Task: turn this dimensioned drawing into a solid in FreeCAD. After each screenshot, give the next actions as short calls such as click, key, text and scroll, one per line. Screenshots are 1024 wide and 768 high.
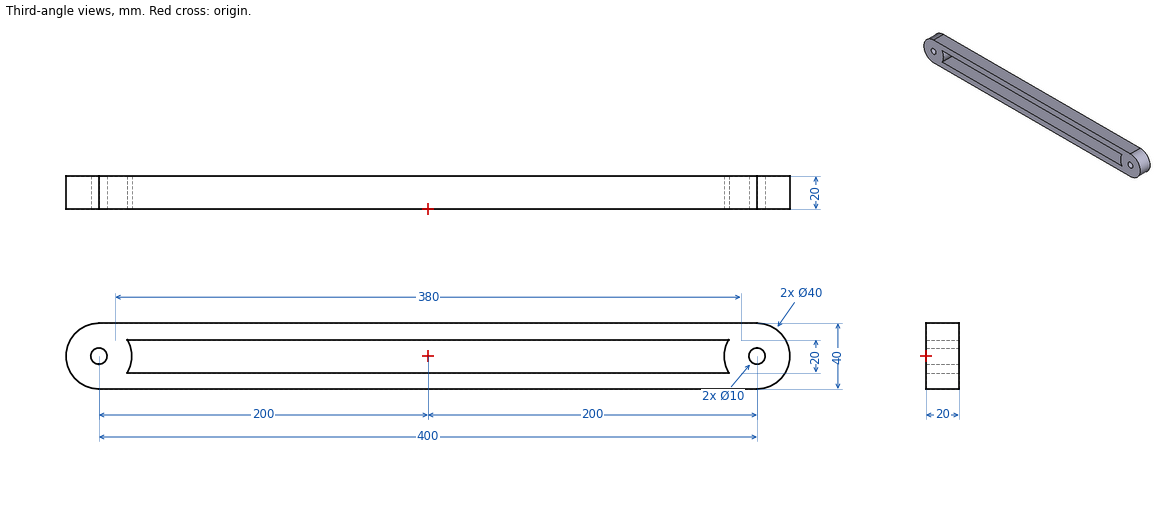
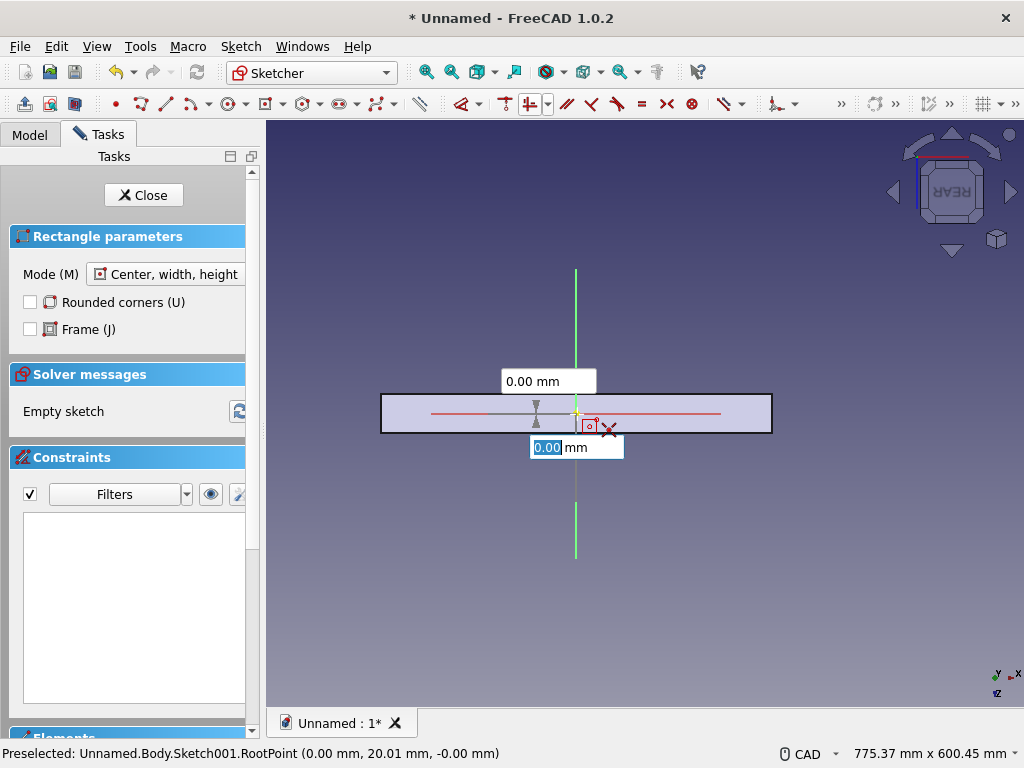
scroll(762, 404, up, 3)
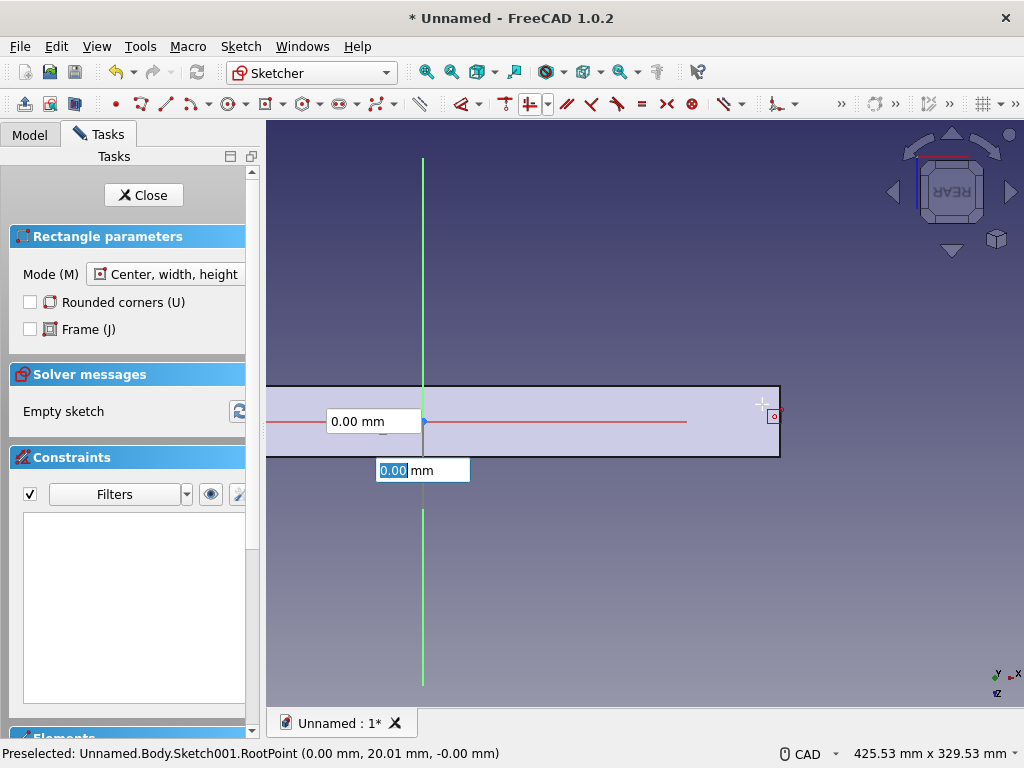
click(762, 404)
key(Escape)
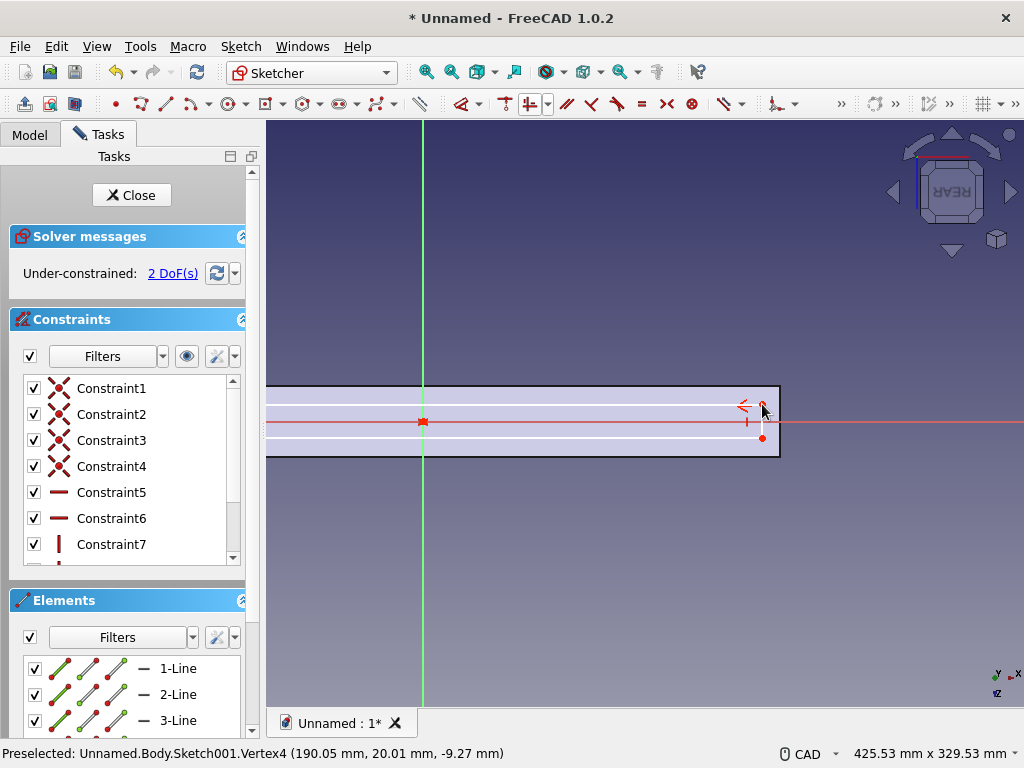
click(460, 104)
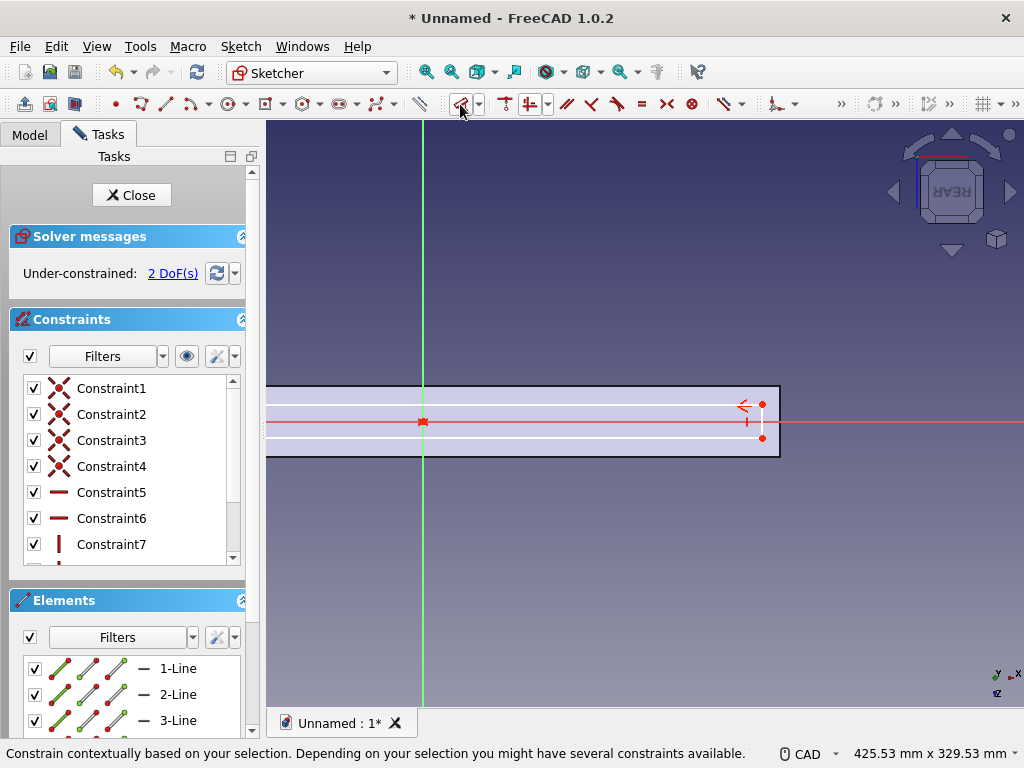
click(762, 425)
click(796, 414)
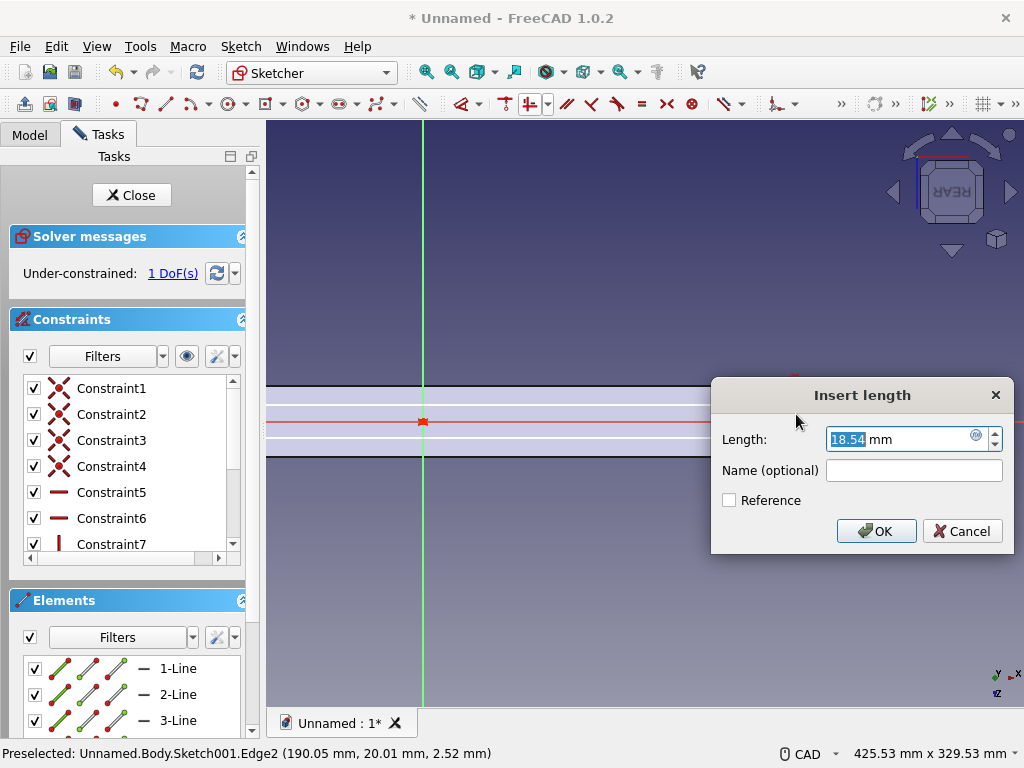
text(20)
key(Return)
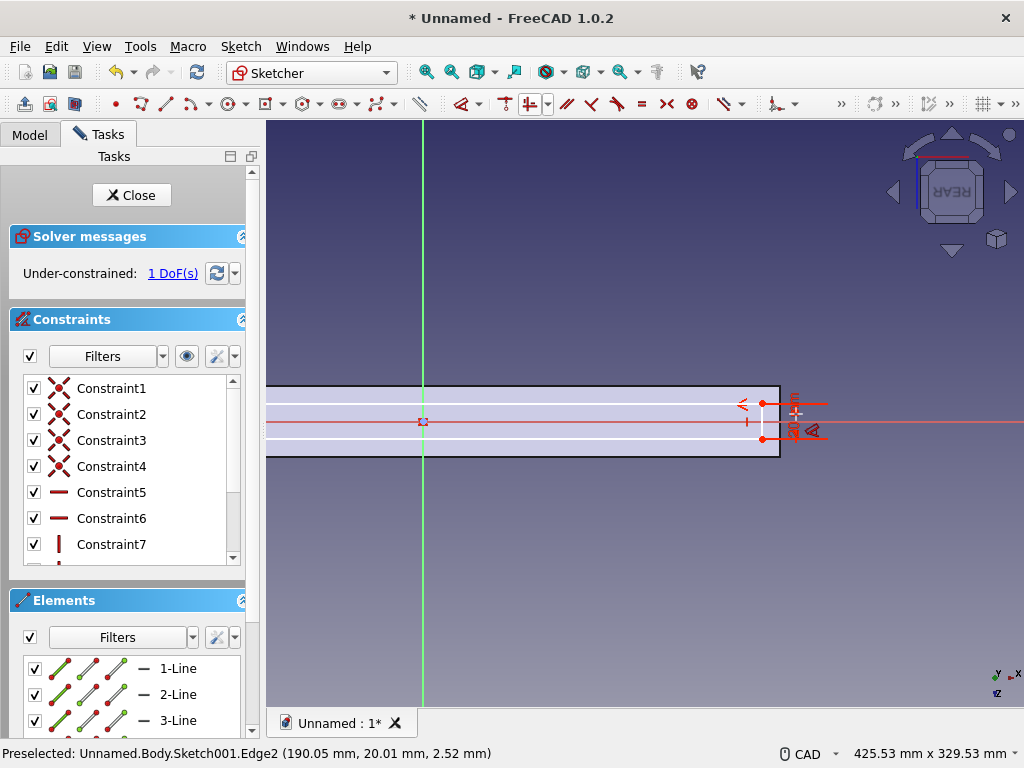
click(559, 439)
click(528, 473)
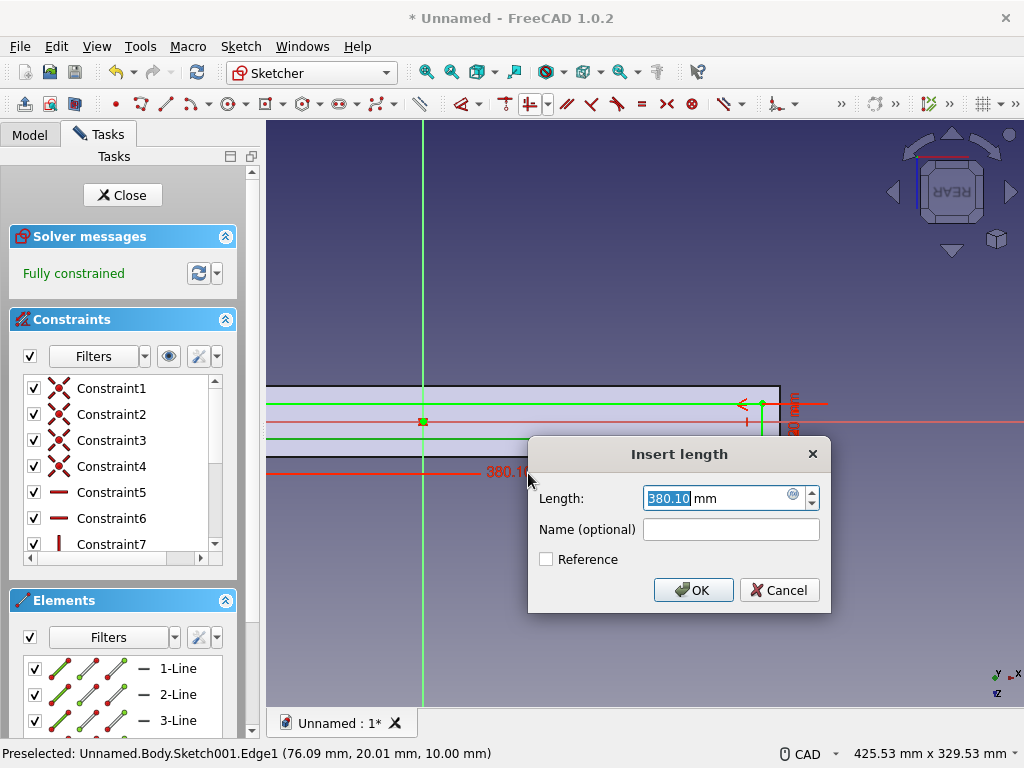
text(380)
key(Return)
key(Escape)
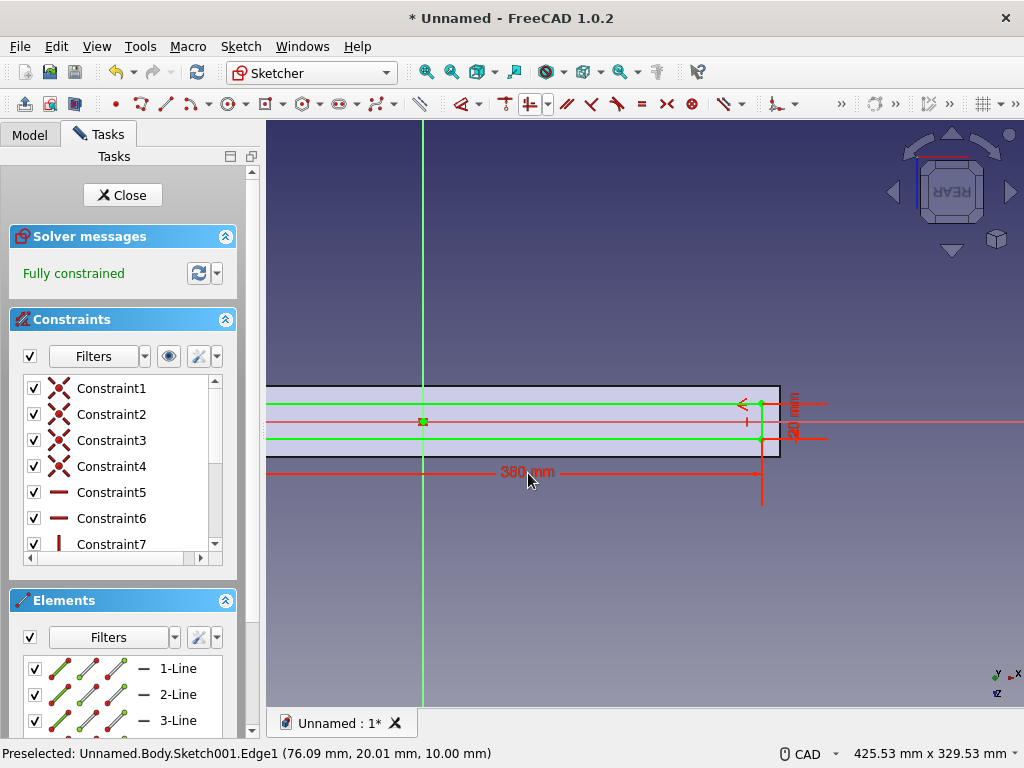
click(123, 195)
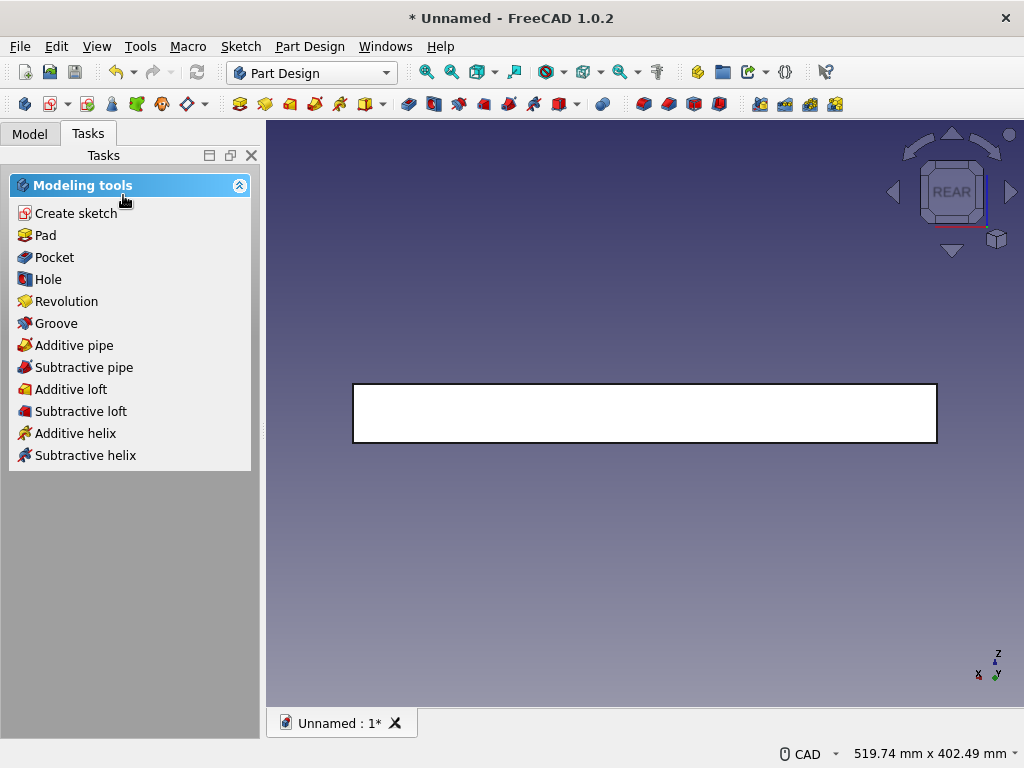
click(409, 104)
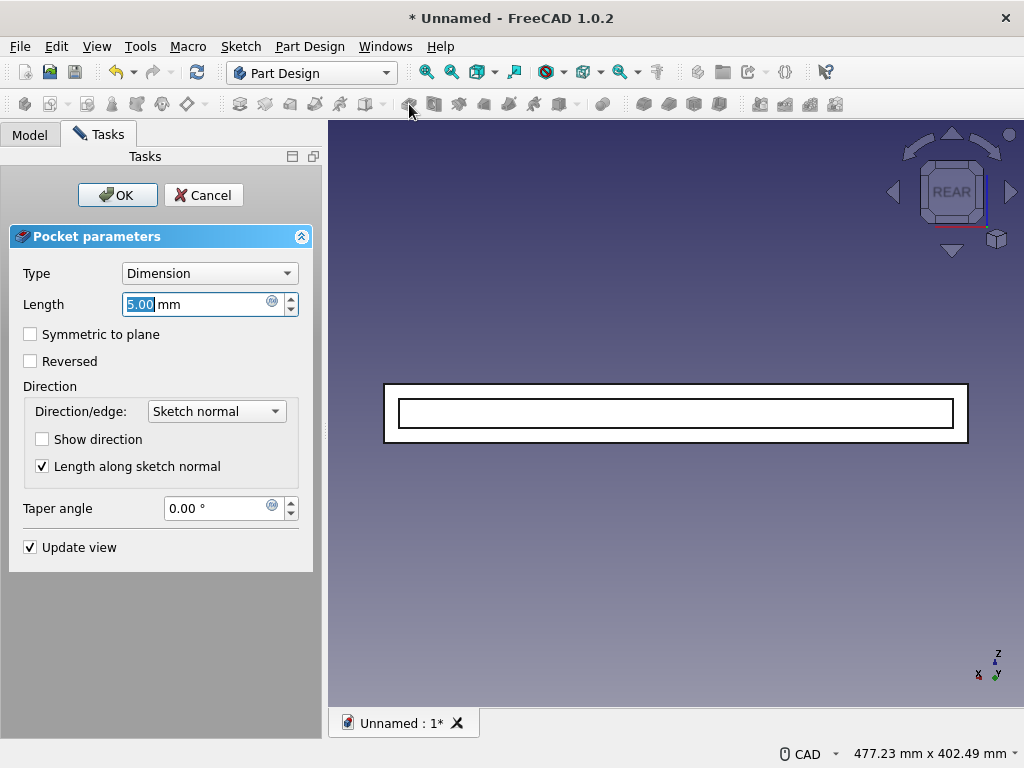
click(210, 274)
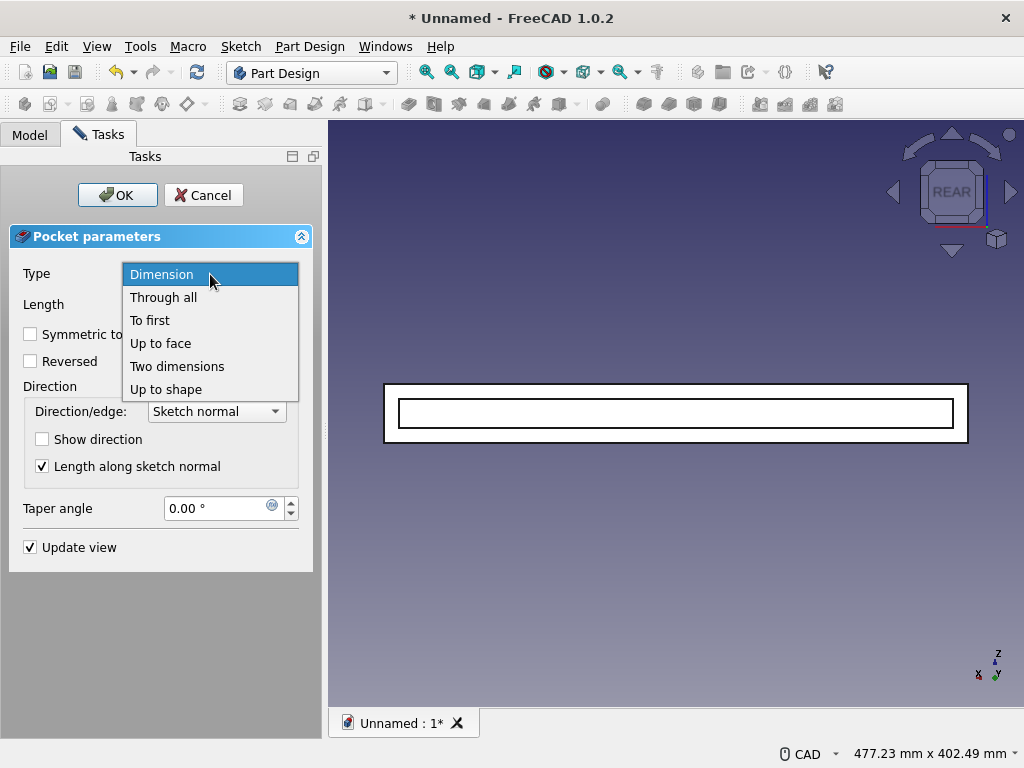
click(208, 298)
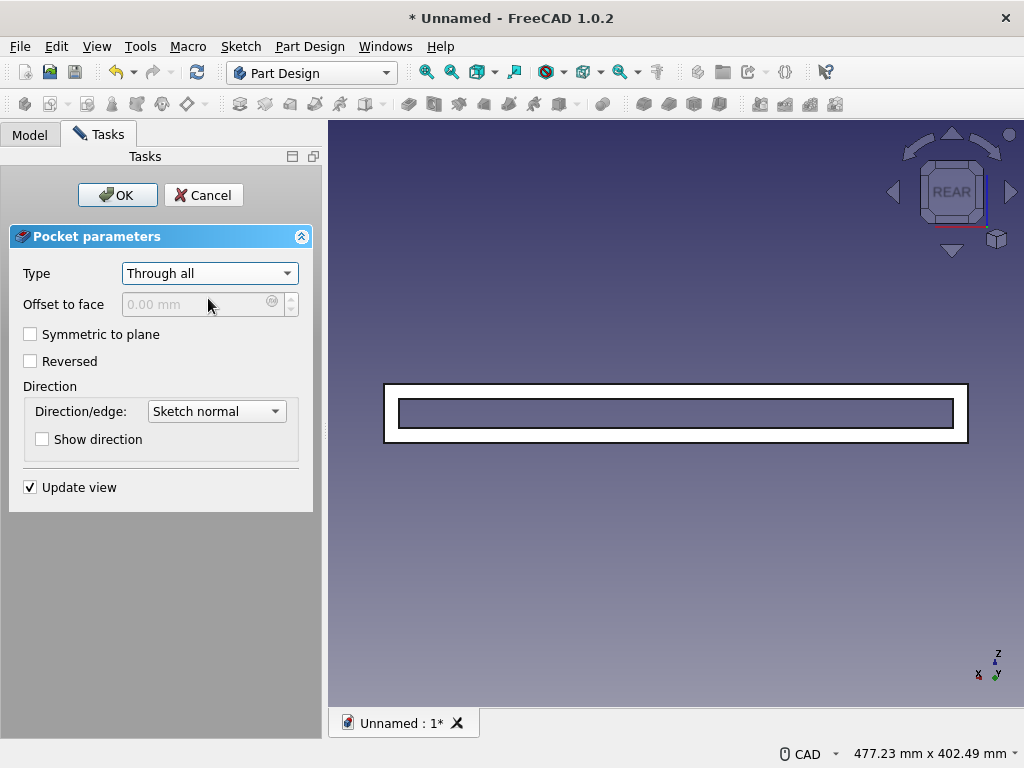
click(118, 195)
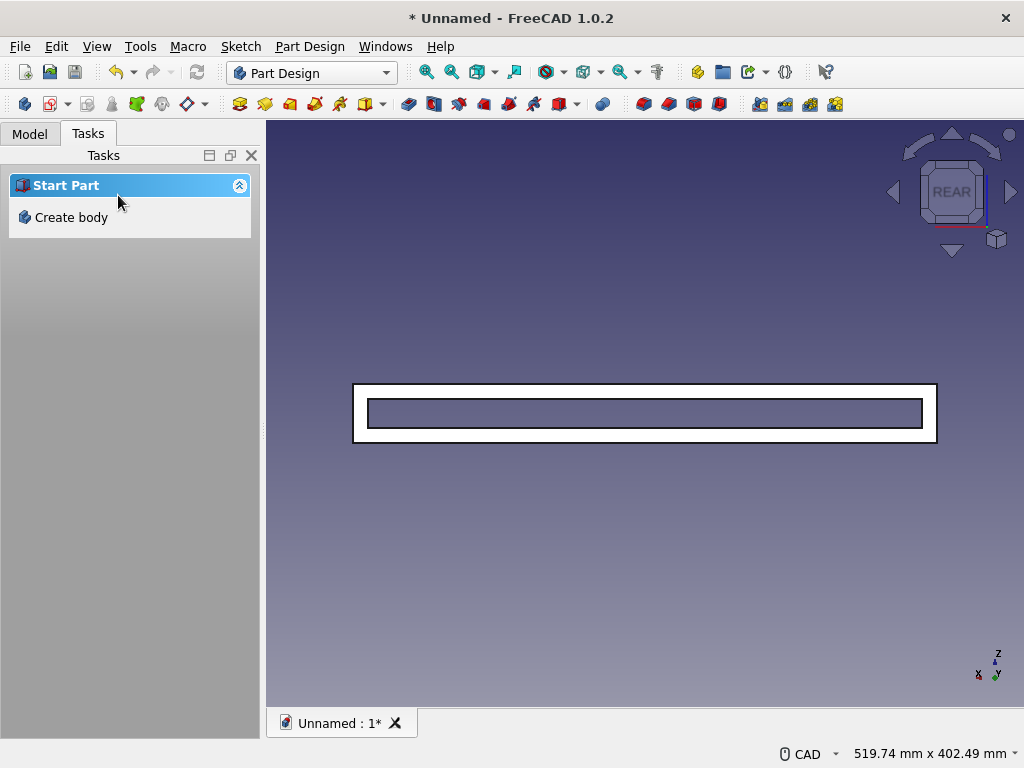
click(395, 387)